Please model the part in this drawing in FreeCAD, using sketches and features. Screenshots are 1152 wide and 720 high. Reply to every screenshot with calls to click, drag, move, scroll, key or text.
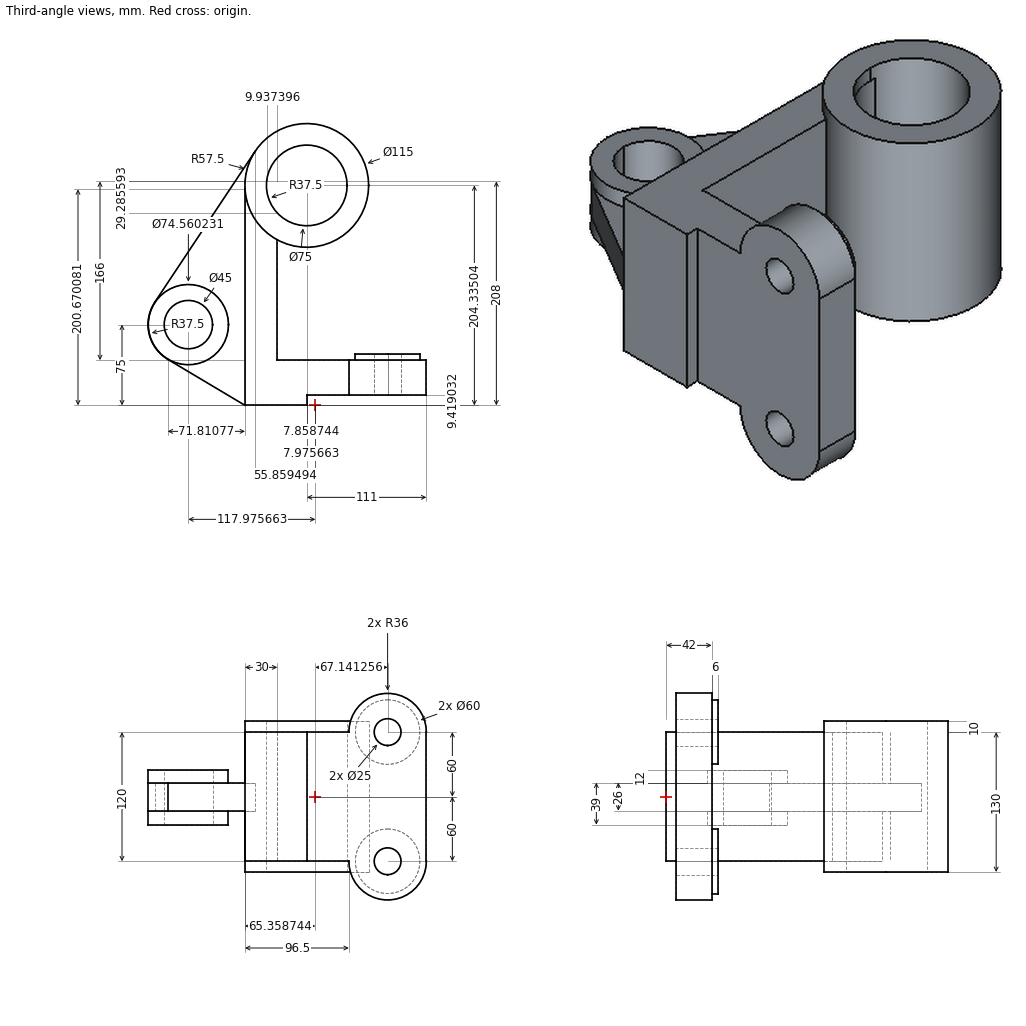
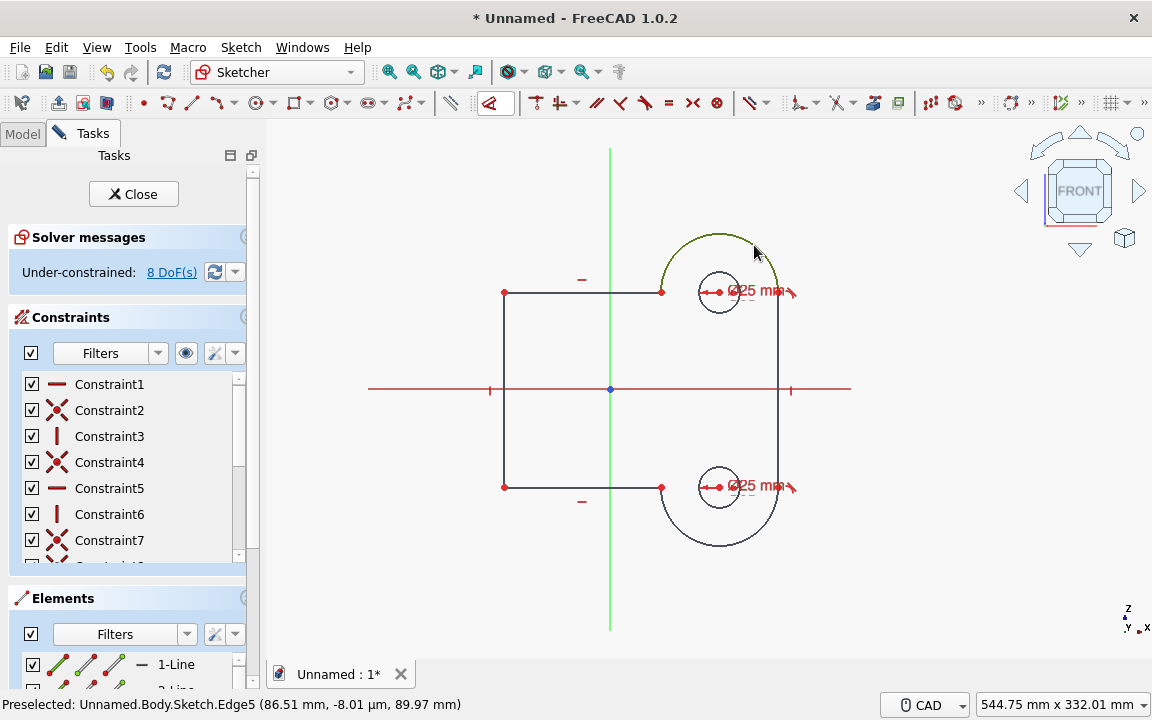
click(685, 535)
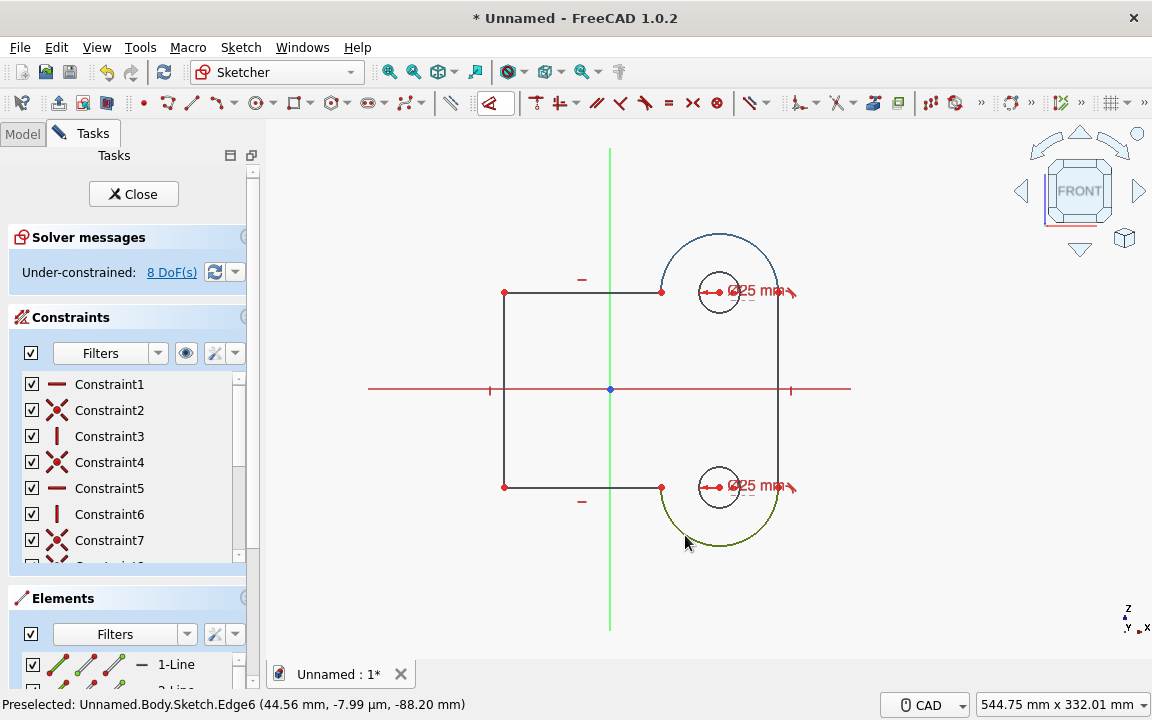
click(670, 104)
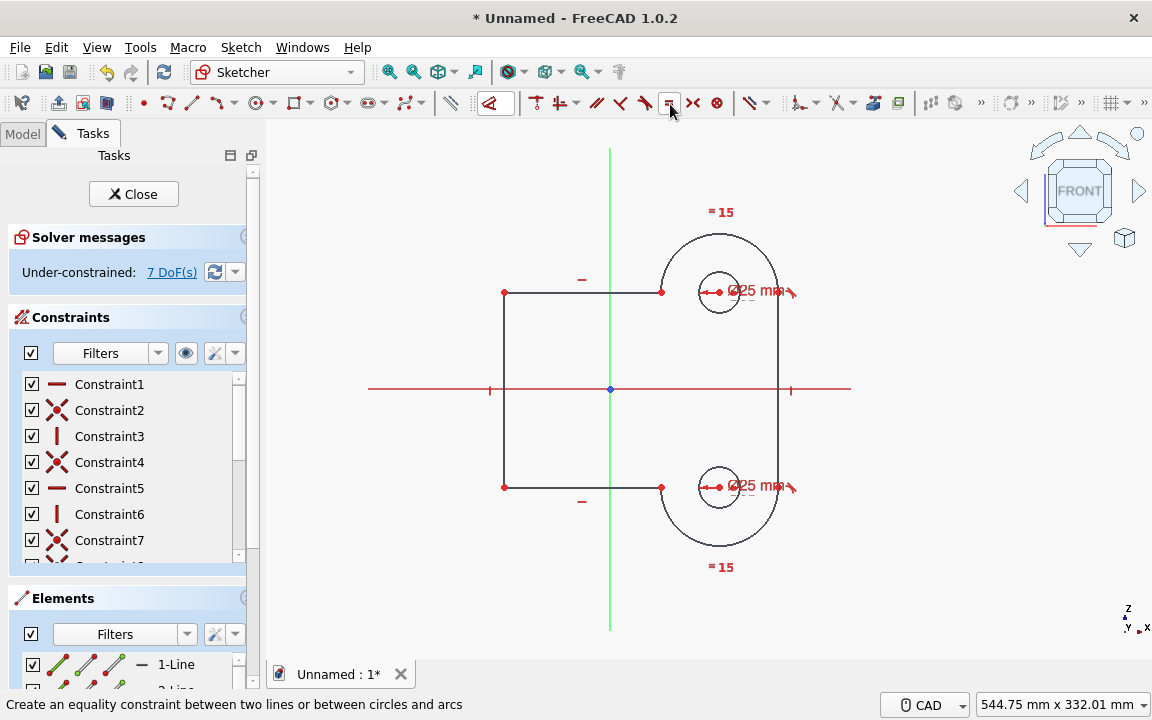
click(490, 104)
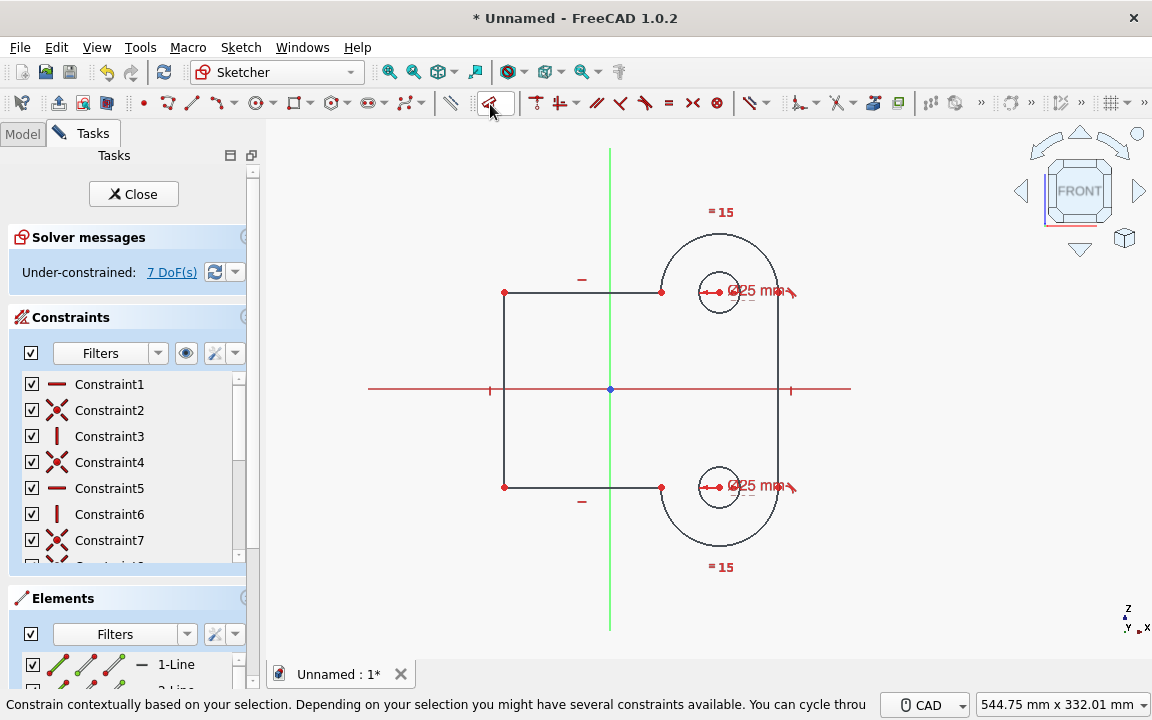
click(754, 245)
click(773, 219)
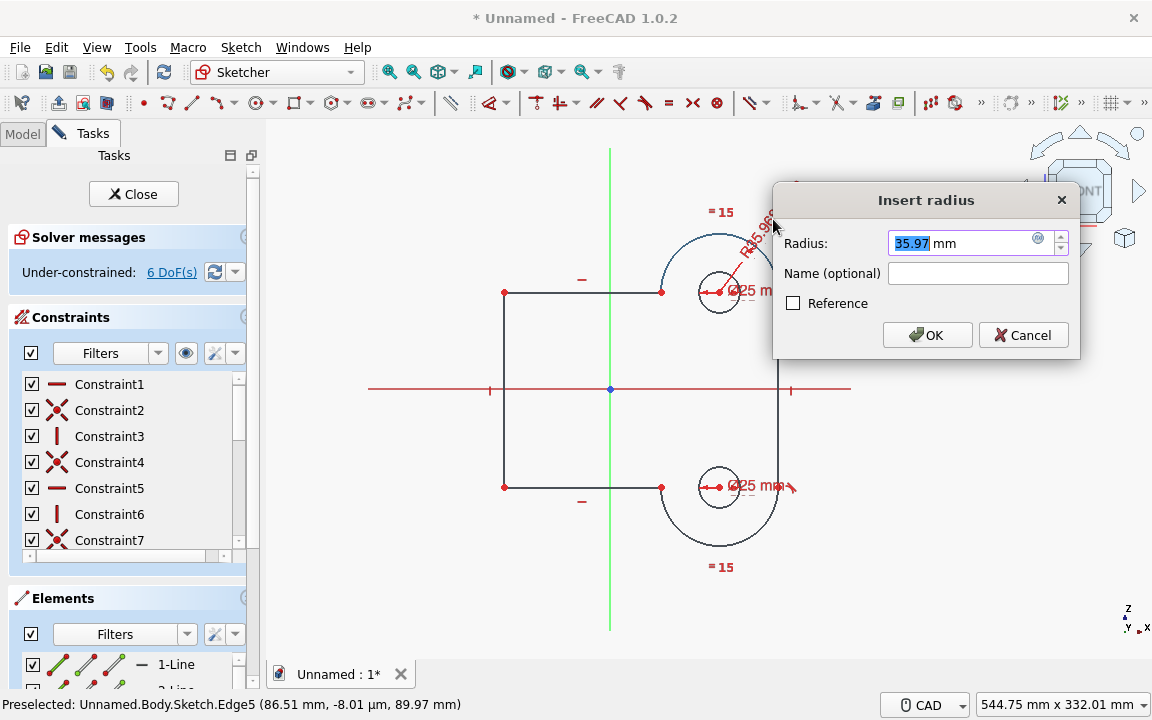
text(36)
key(Return)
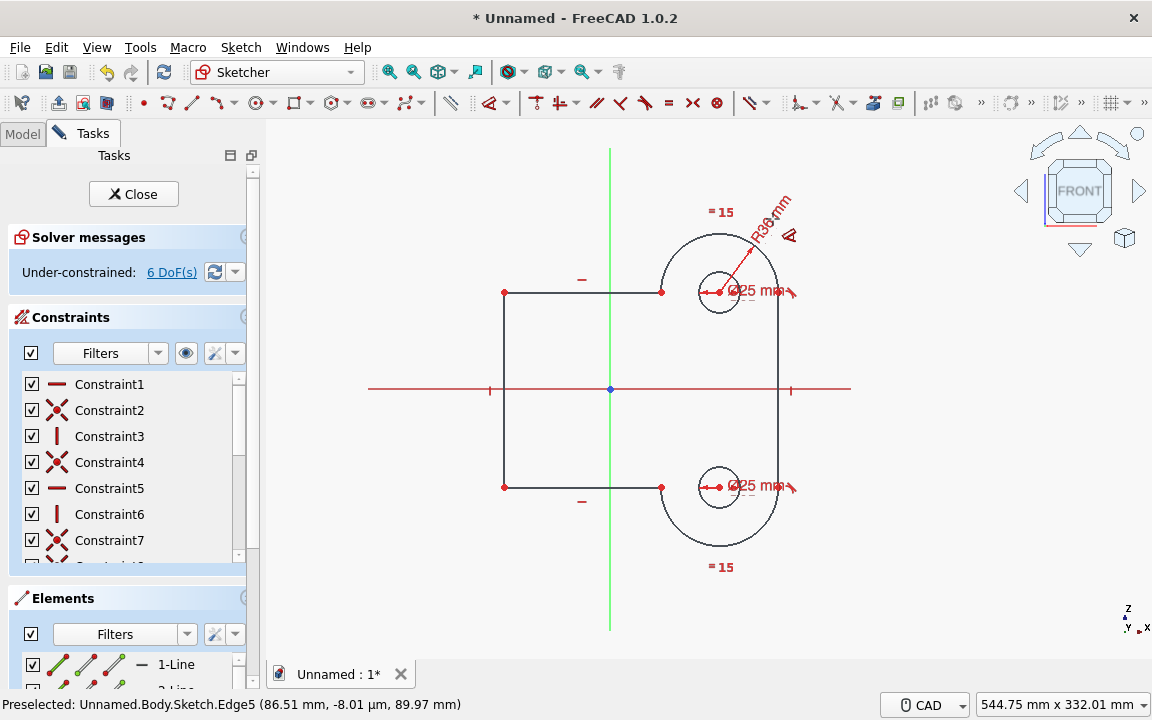
click(720, 293)
click(754, 341)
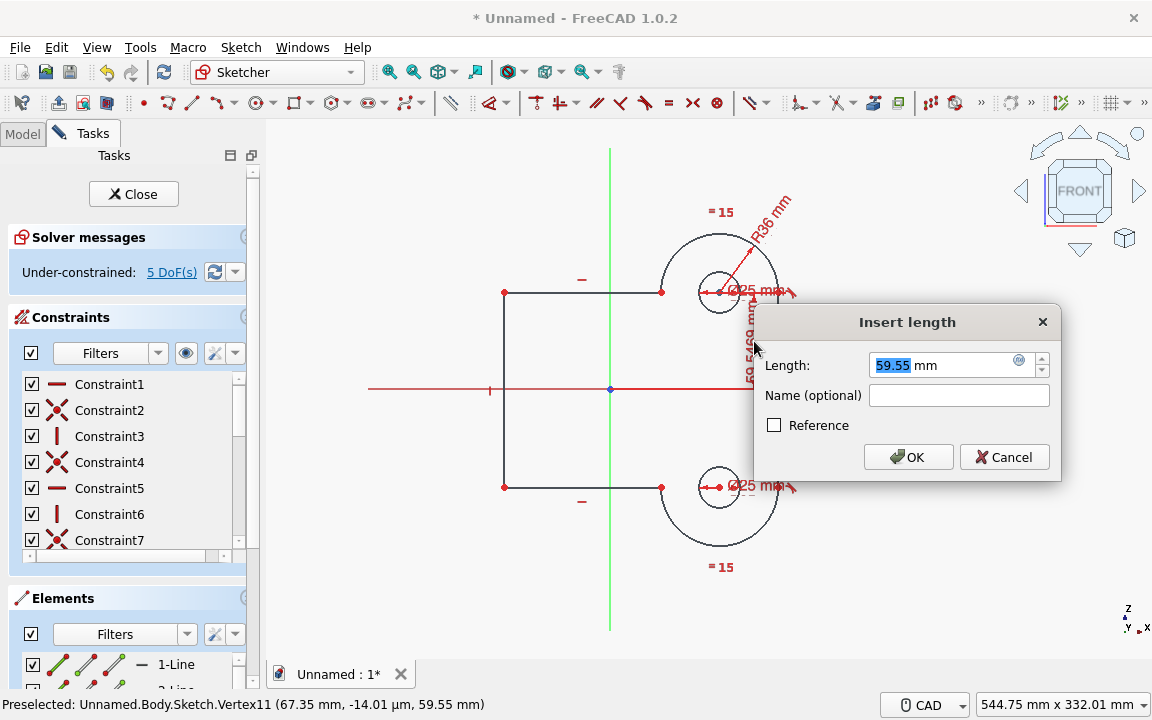
text(60)
key(Return)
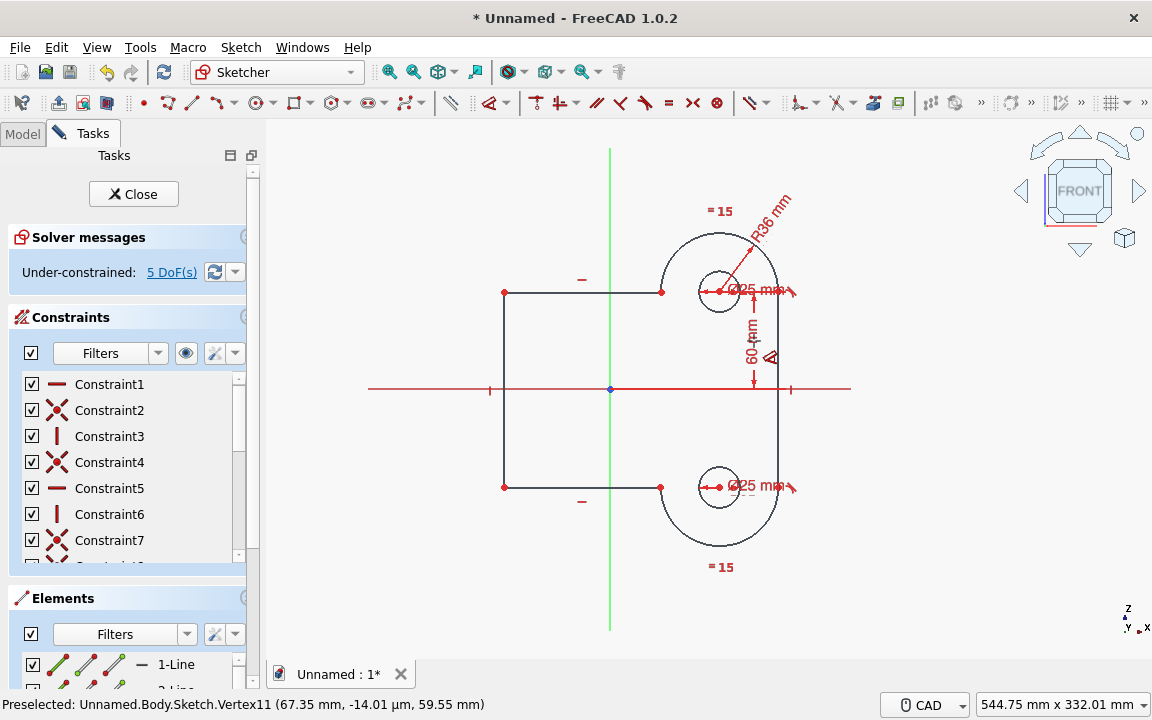
click(720, 488)
click(754, 438)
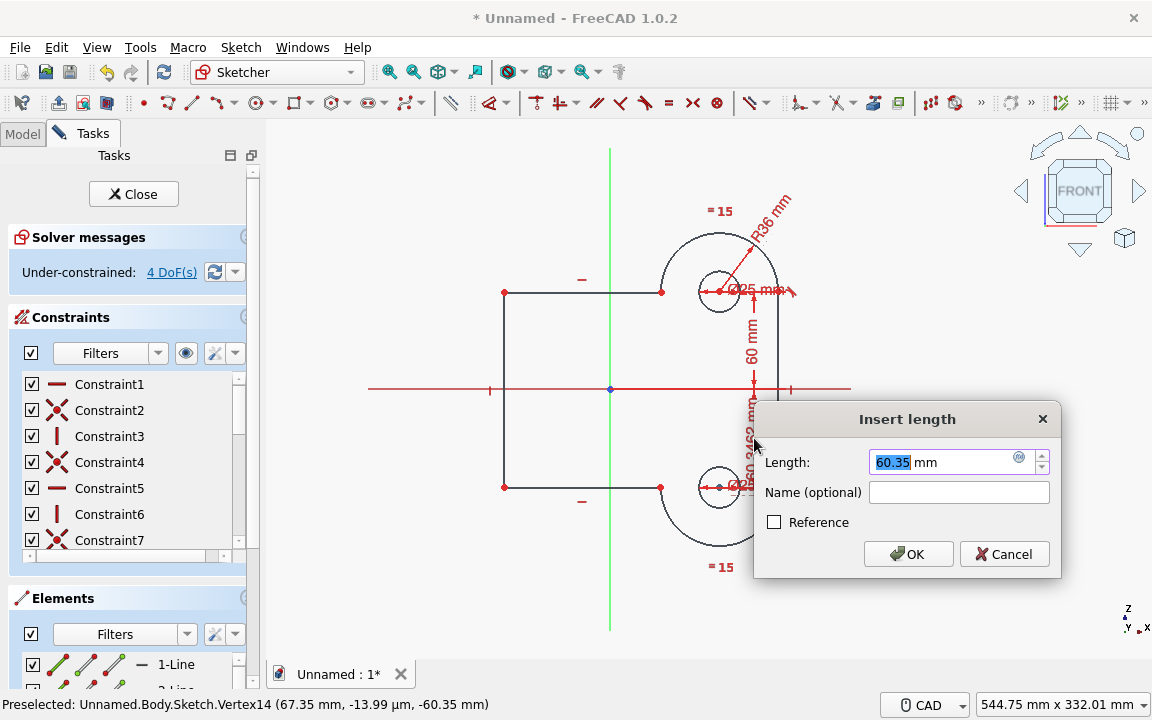
text(60)
key(Return)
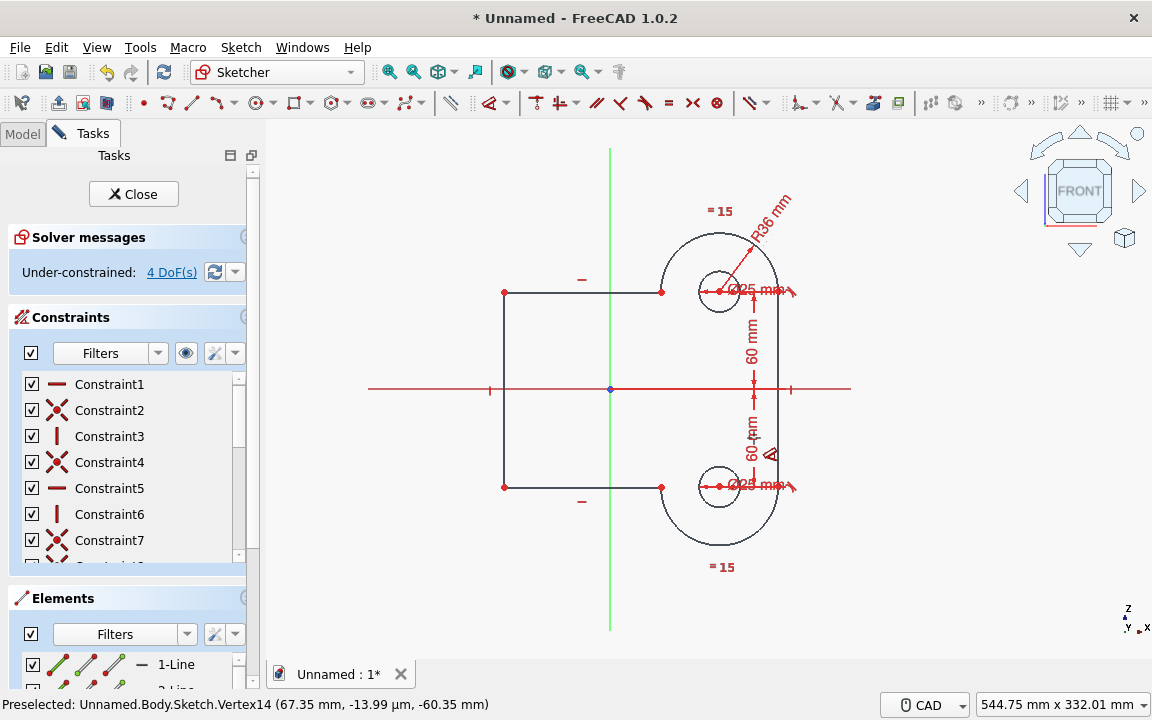
click(504, 429)
click(470, 346)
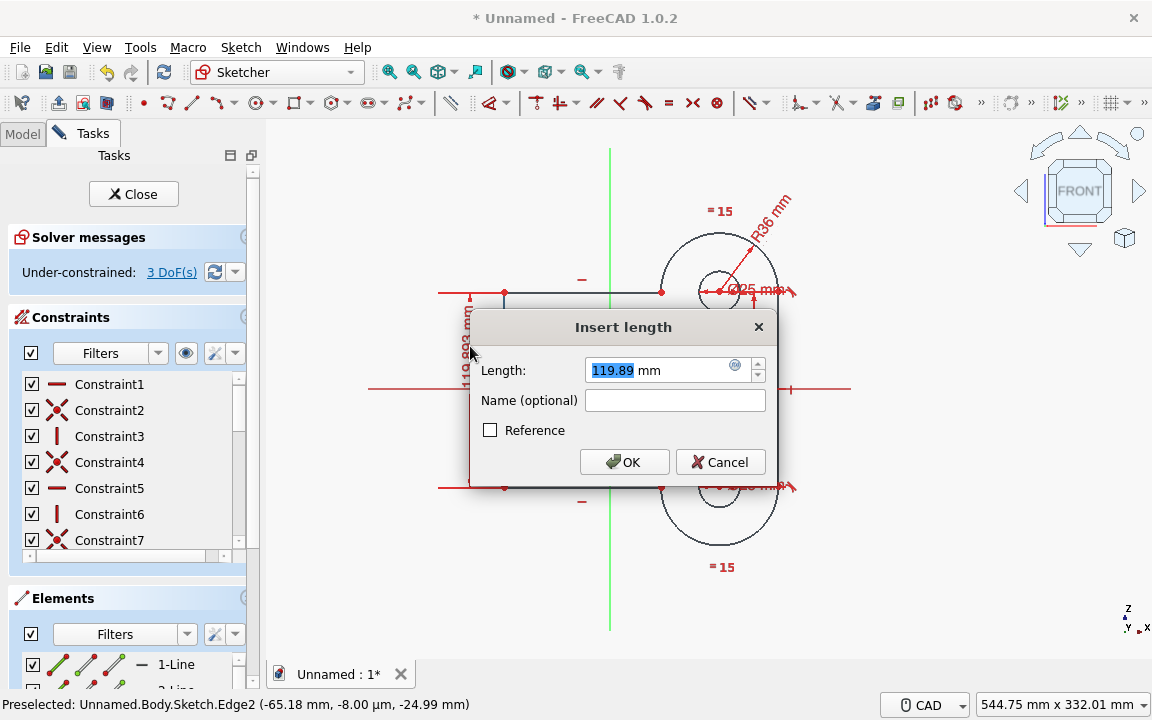
text(120)
key(Return)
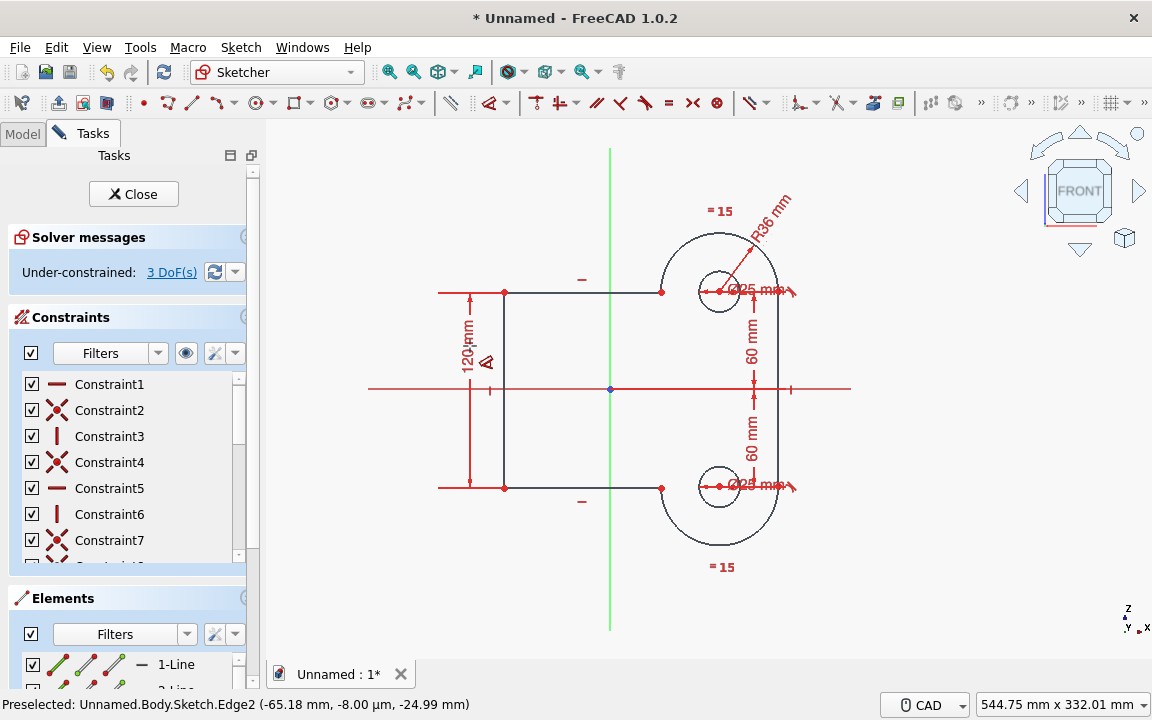
click(661, 488)
click(576, 439)